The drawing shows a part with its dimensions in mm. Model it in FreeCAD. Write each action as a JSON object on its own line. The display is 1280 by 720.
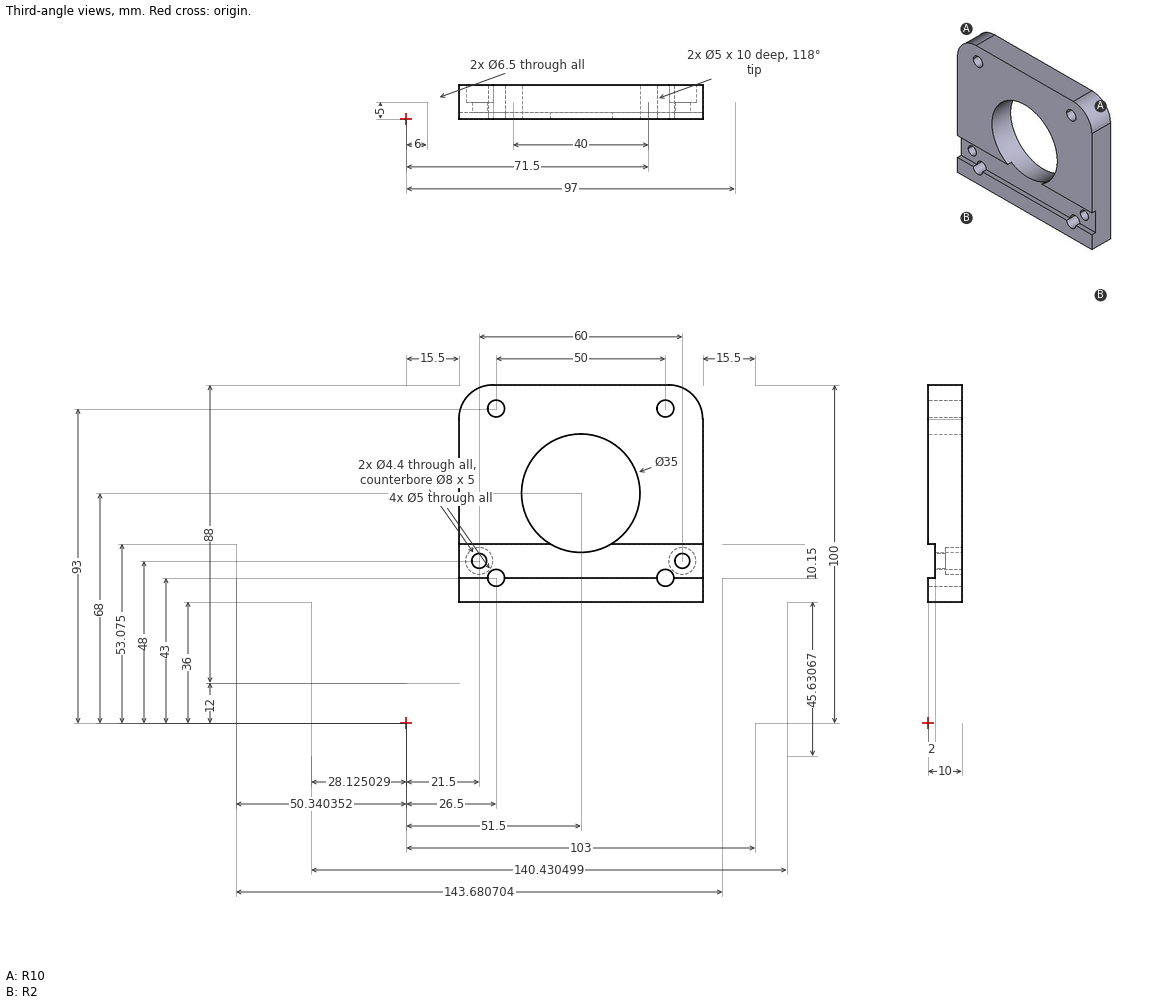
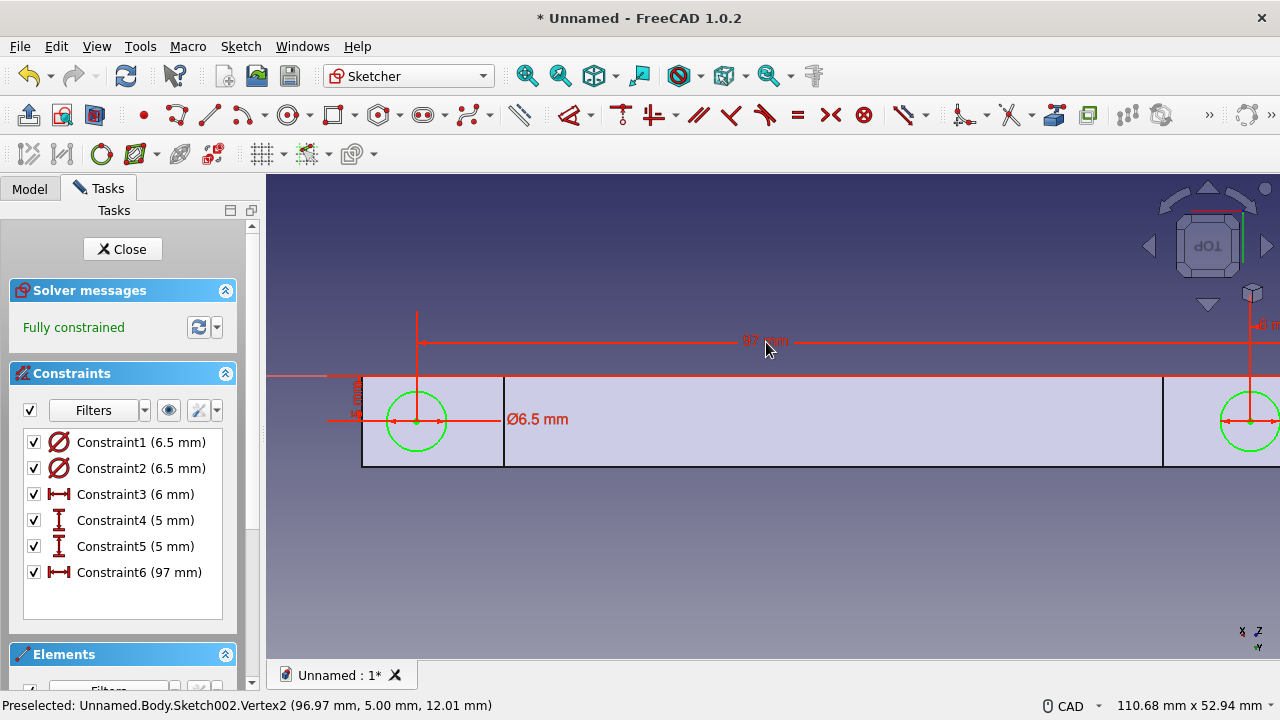
{"action": "left_click", "coordinate": [123, 249]}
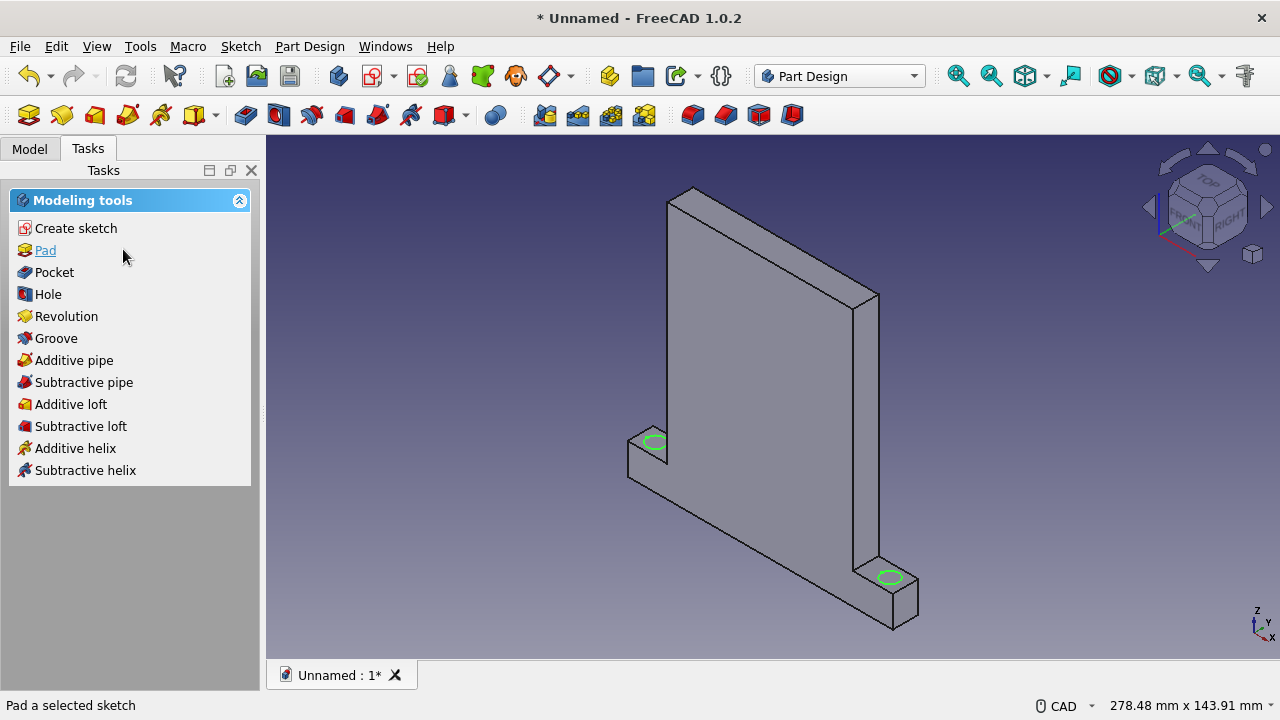
{"action": "left_click", "coordinate": [279, 116]}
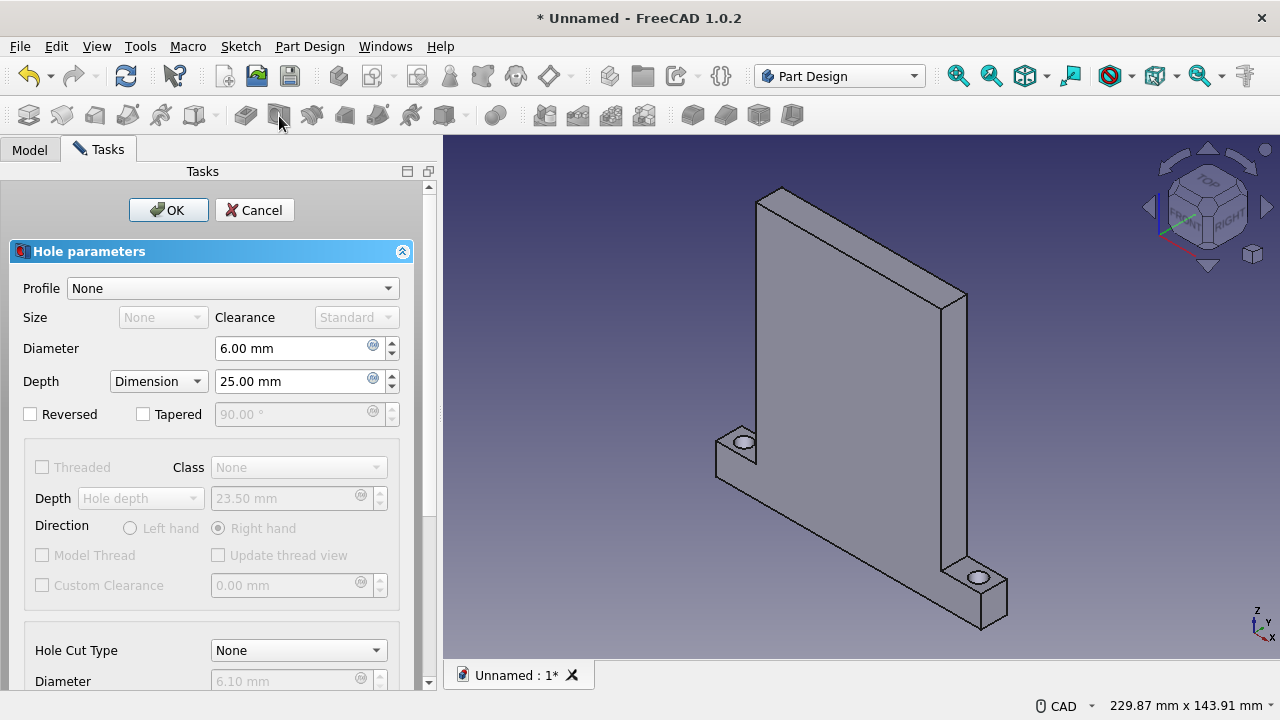
{"action": "triple_click", "coordinate": [300, 348]}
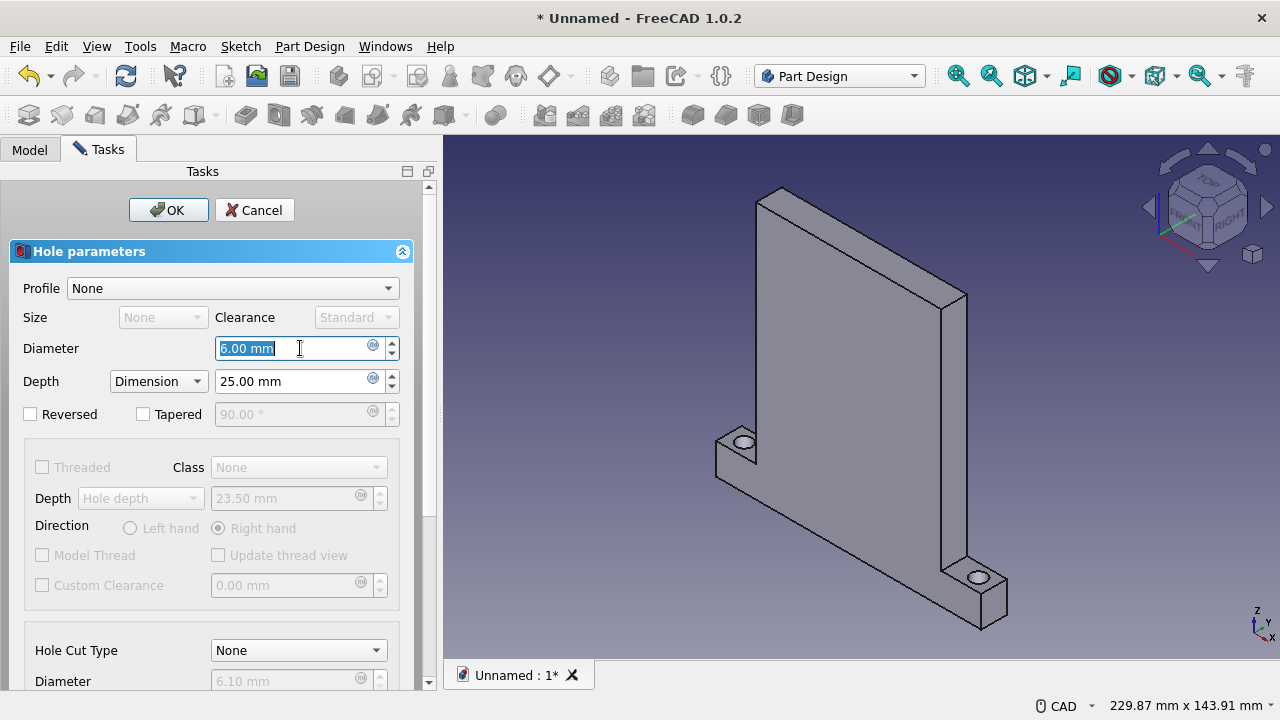
{"action": "type", "text": "6.5"}
{"action": "key", "text": "Tab"}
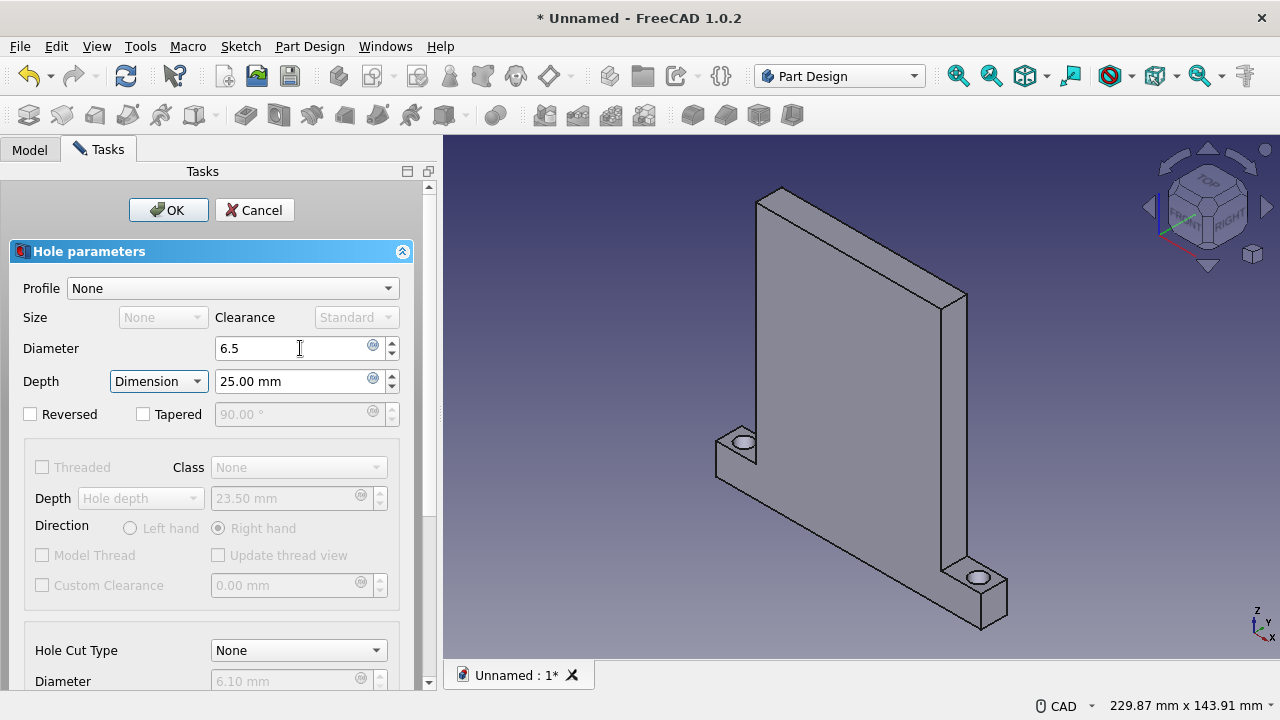
{"action": "left_click", "coordinate": [160, 382]}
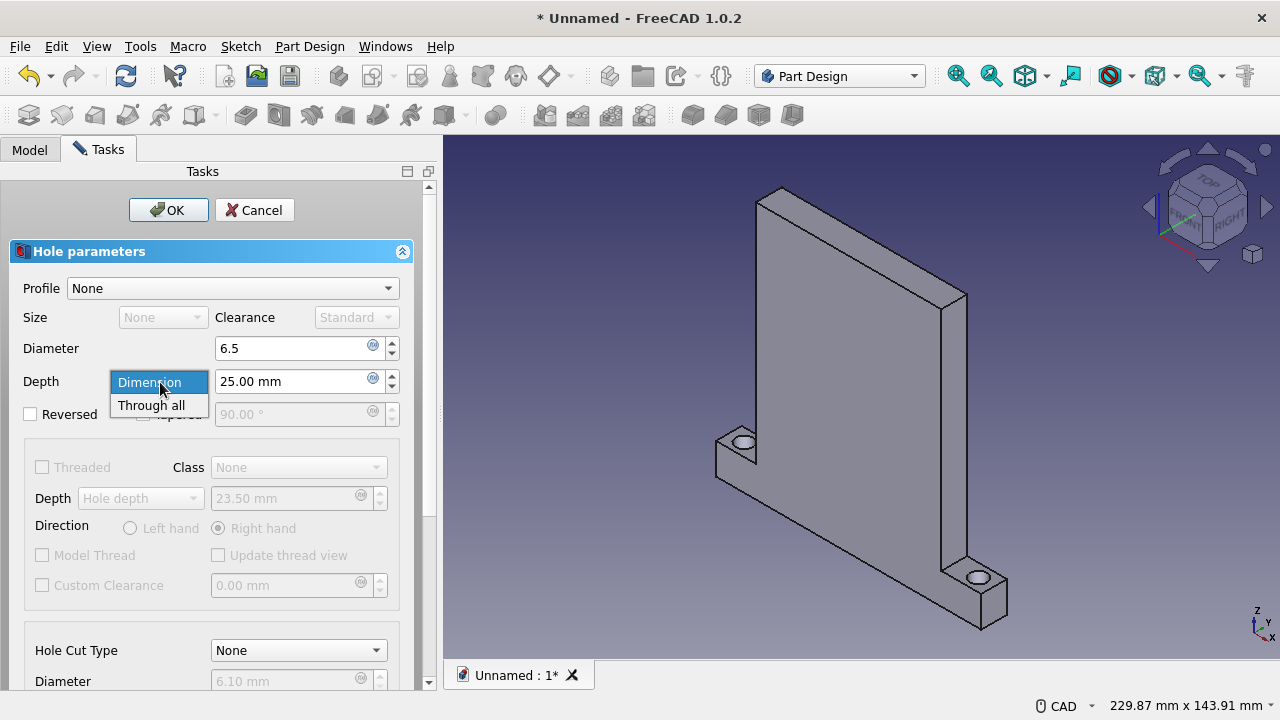
{"action": "left_click", "coordinate": [158, 406]}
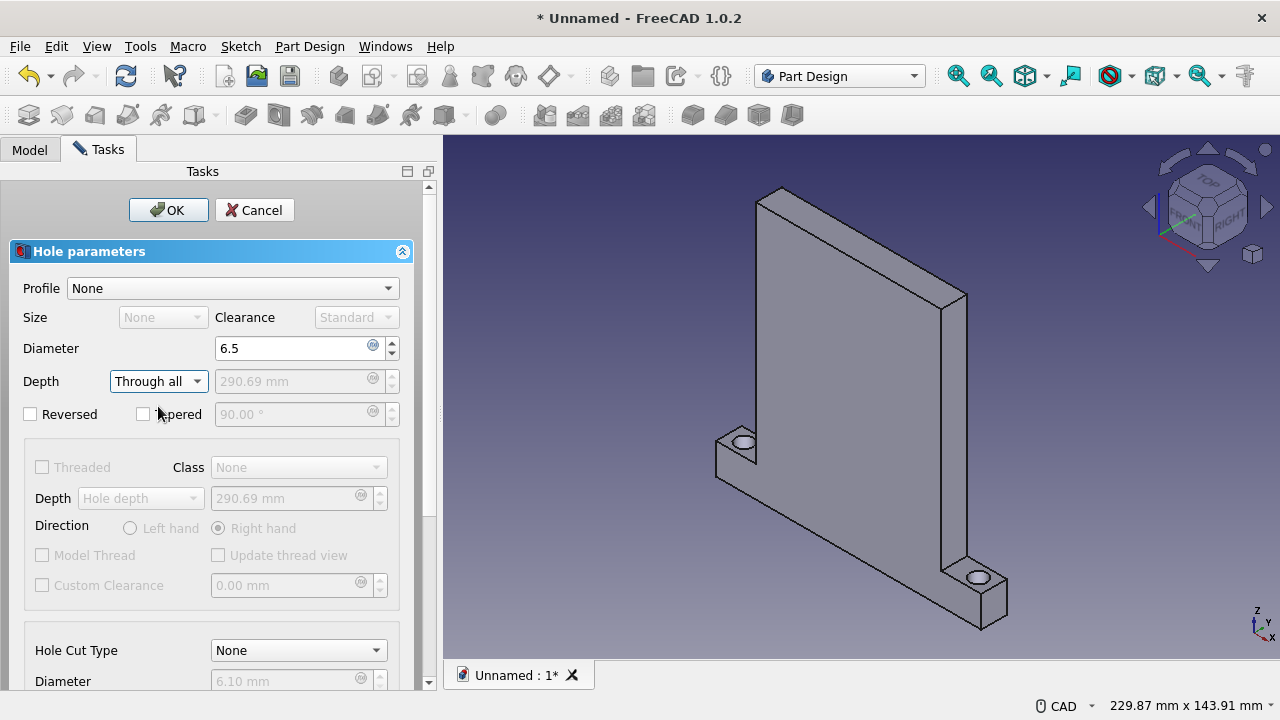
{"action": "left_click", "coordinate": [169, 210]}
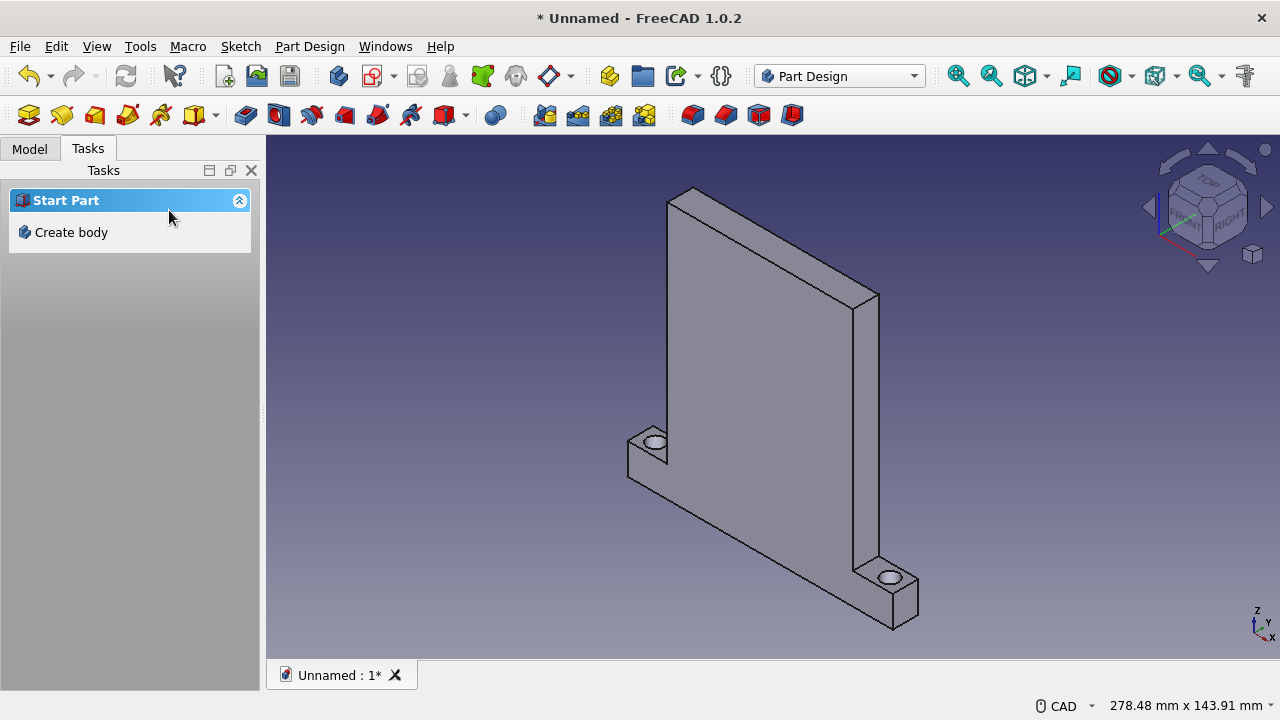
{"action": "key", "text": "4"}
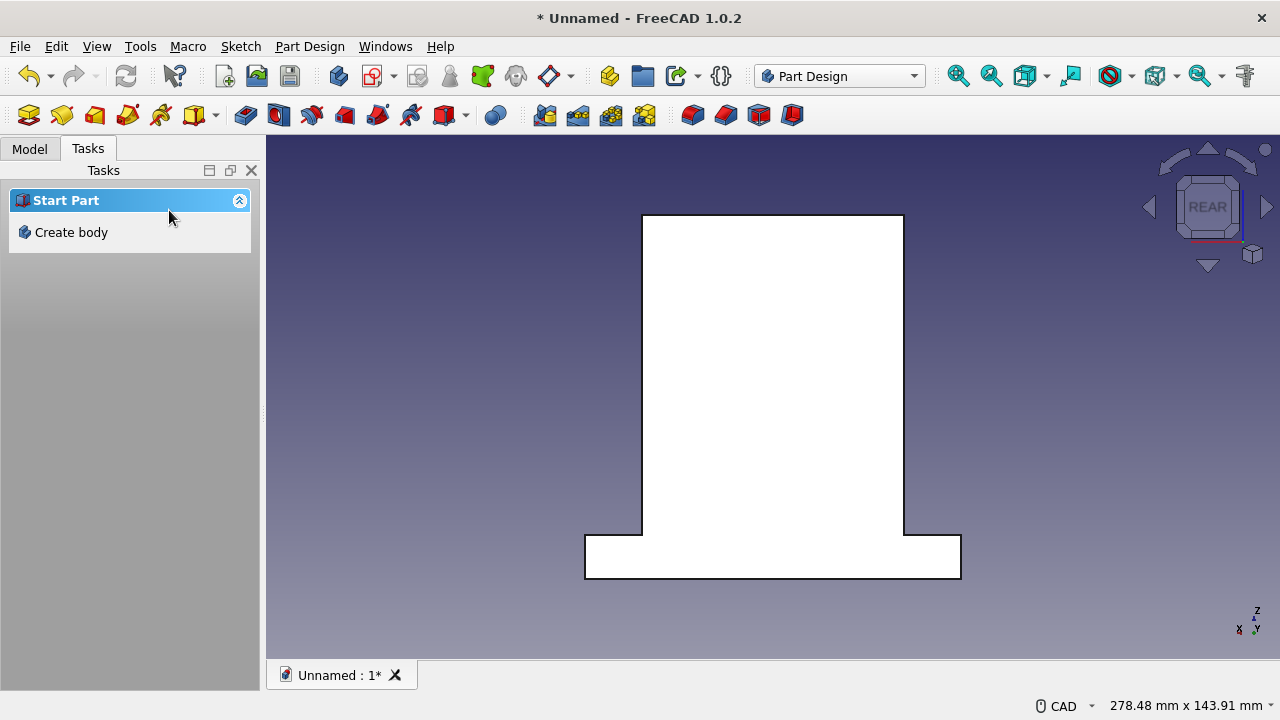
{"action": "left_click", "coordinate": [773, 396]}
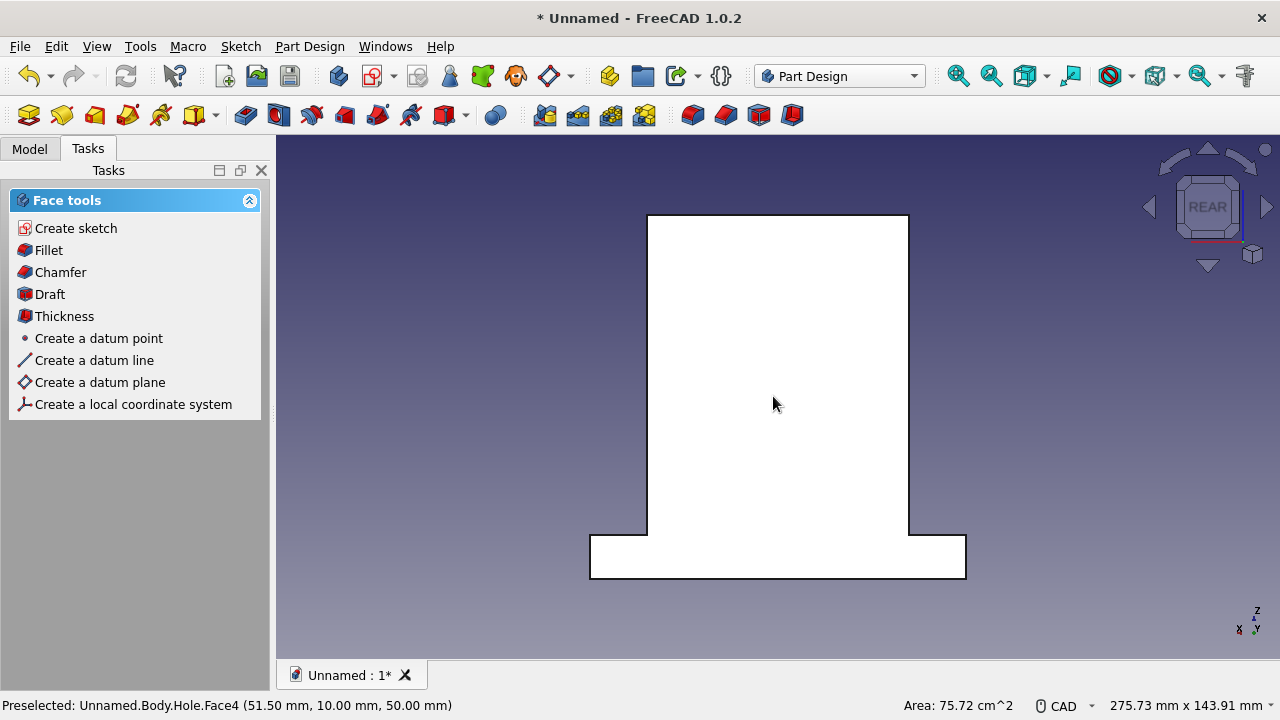
{"action": "left_click", "coordinate": [372, 76]}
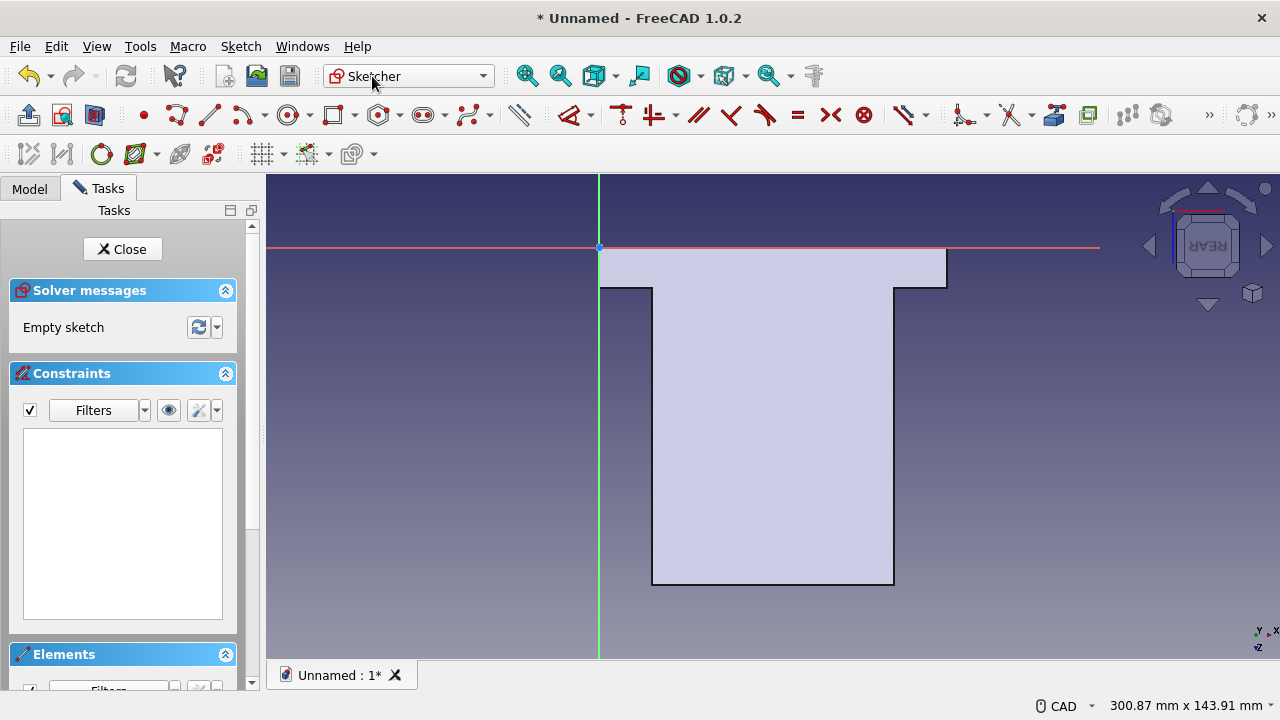
{"action": "left_click", "coordinate": [288, 116]}